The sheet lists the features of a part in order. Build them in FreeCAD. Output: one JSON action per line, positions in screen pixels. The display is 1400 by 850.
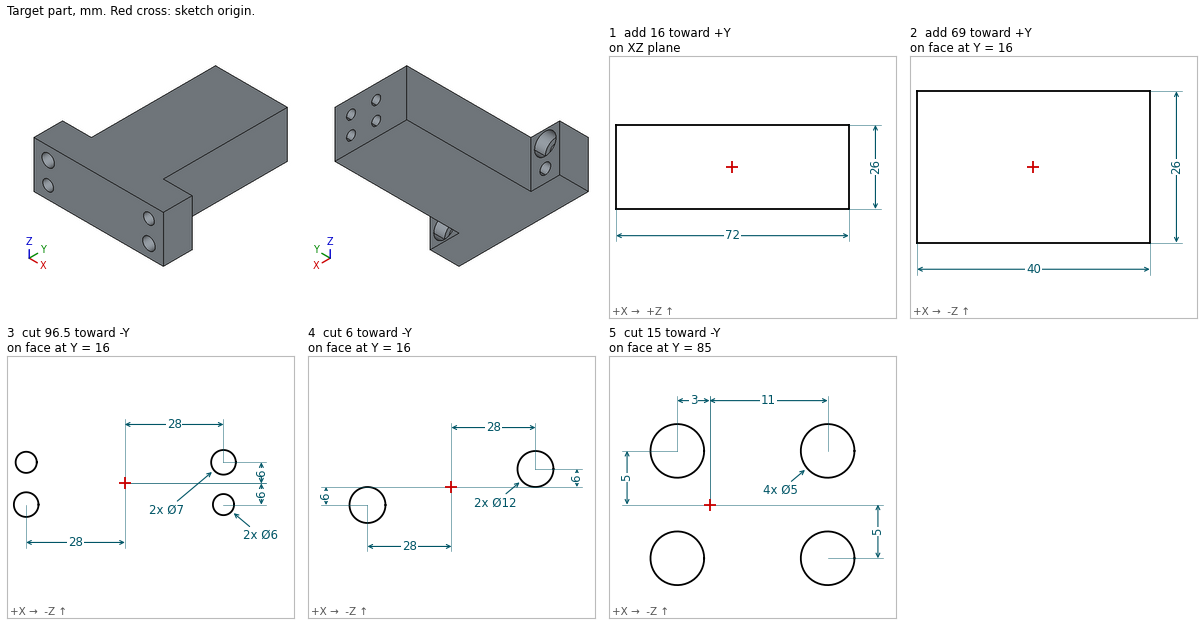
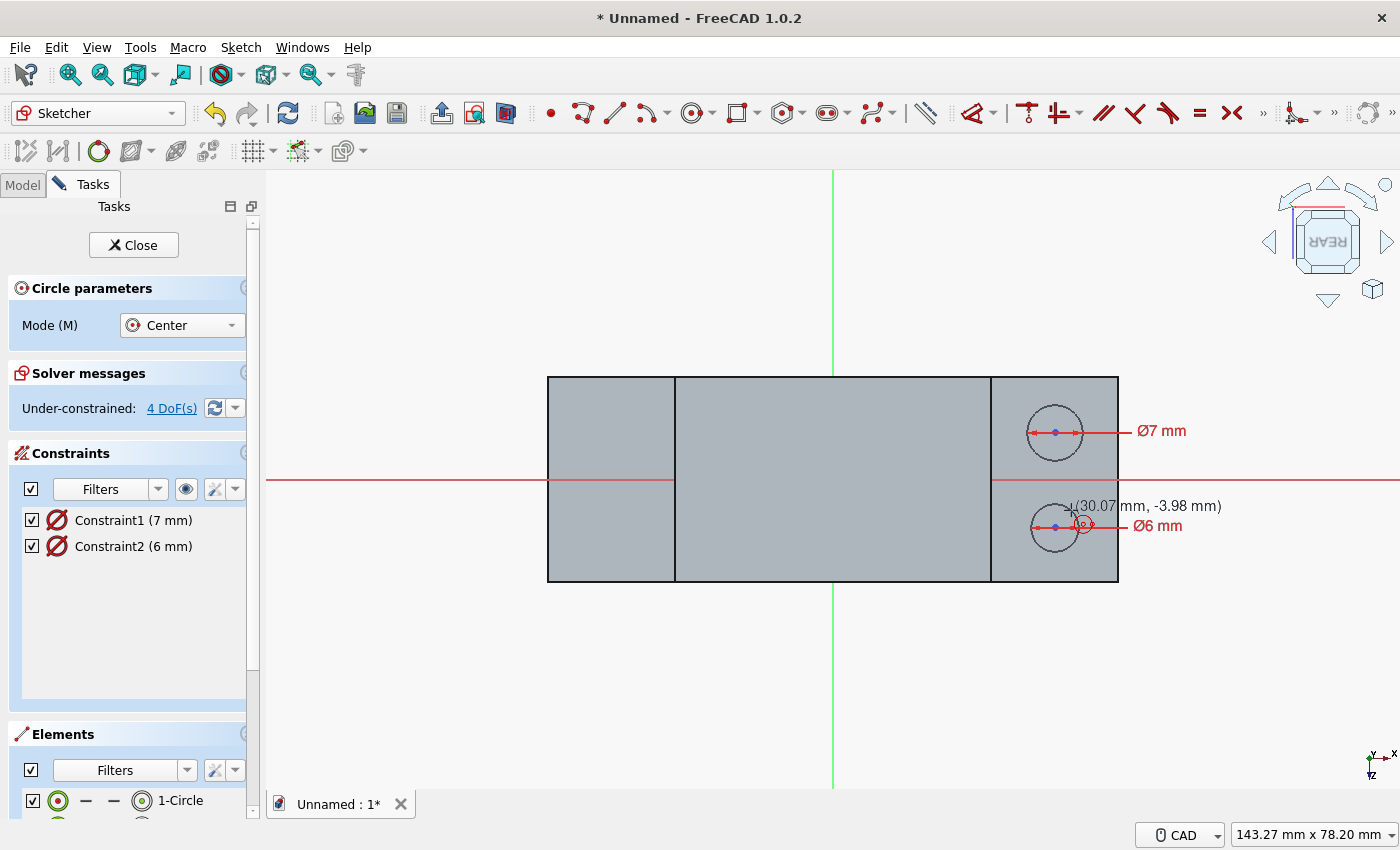
{"action": "left_click", "coordinate": [611, 527]}
{"action": "mouse_move", "coordinate": [631, 507]}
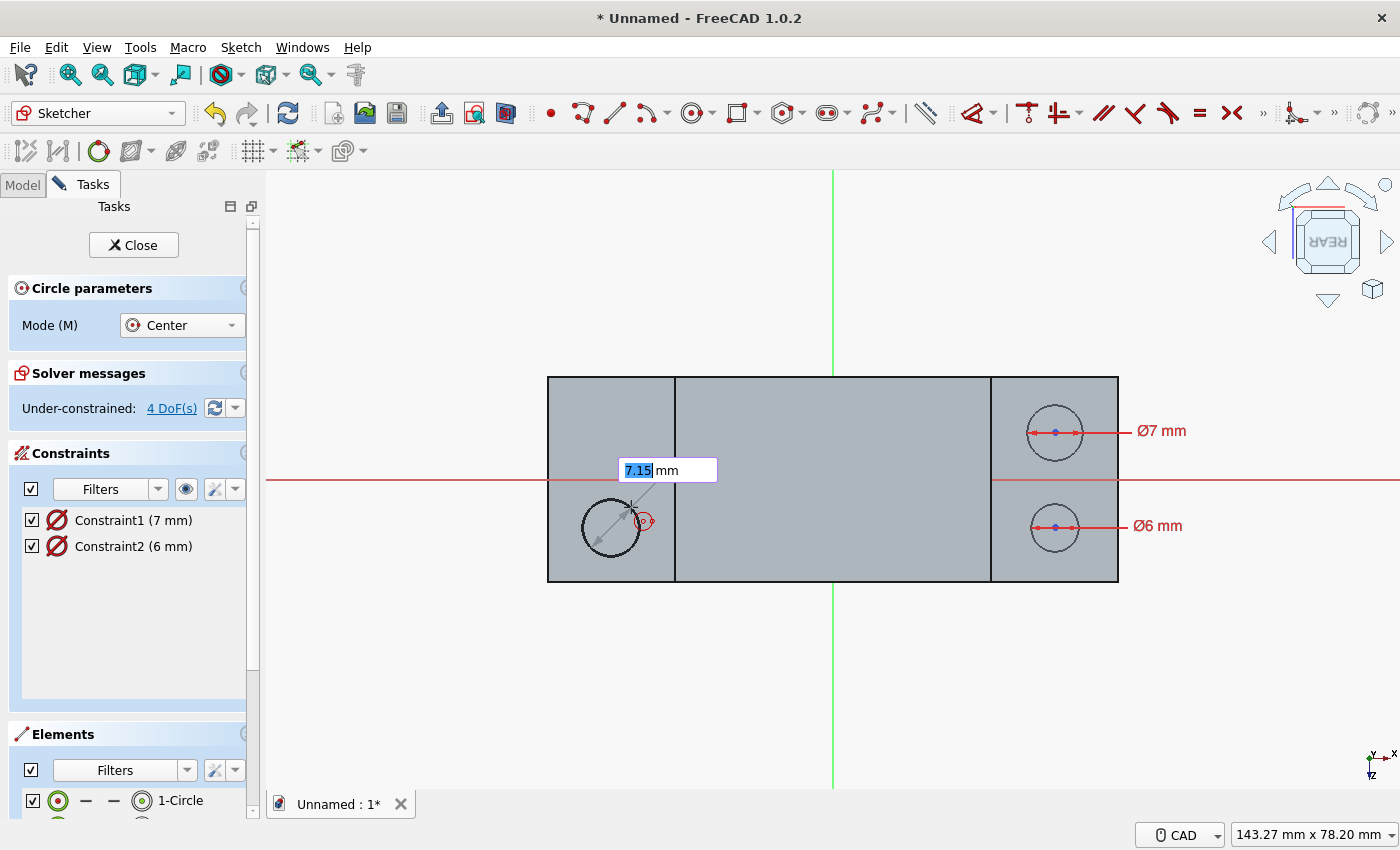
{"action": "type", "text": "7"}
{"action": "key", "text": "Return"}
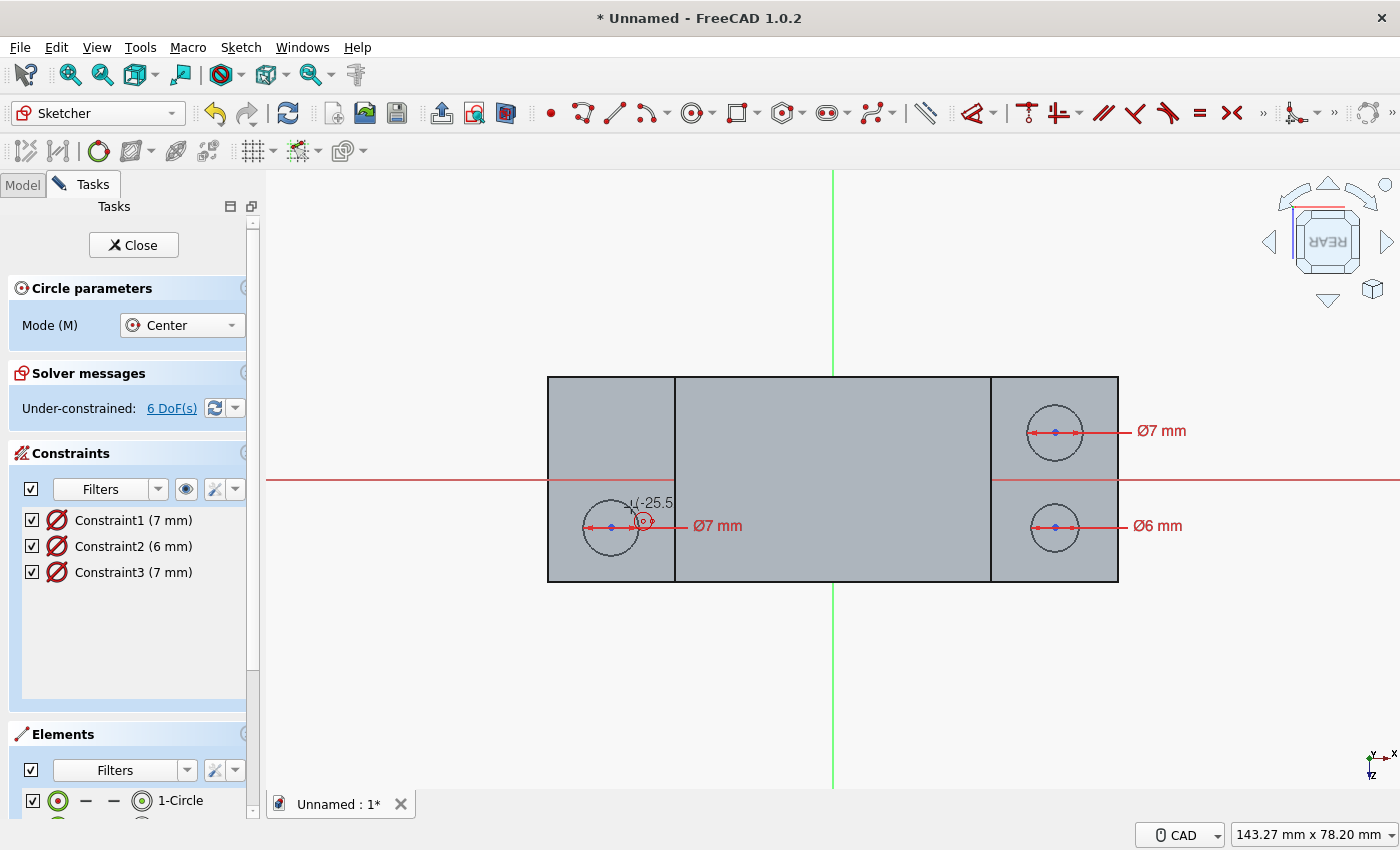
{"action": "left_click", "coordinate": [611, 432]}
{"action": "mouse_move", "coordinate": [628, 415]}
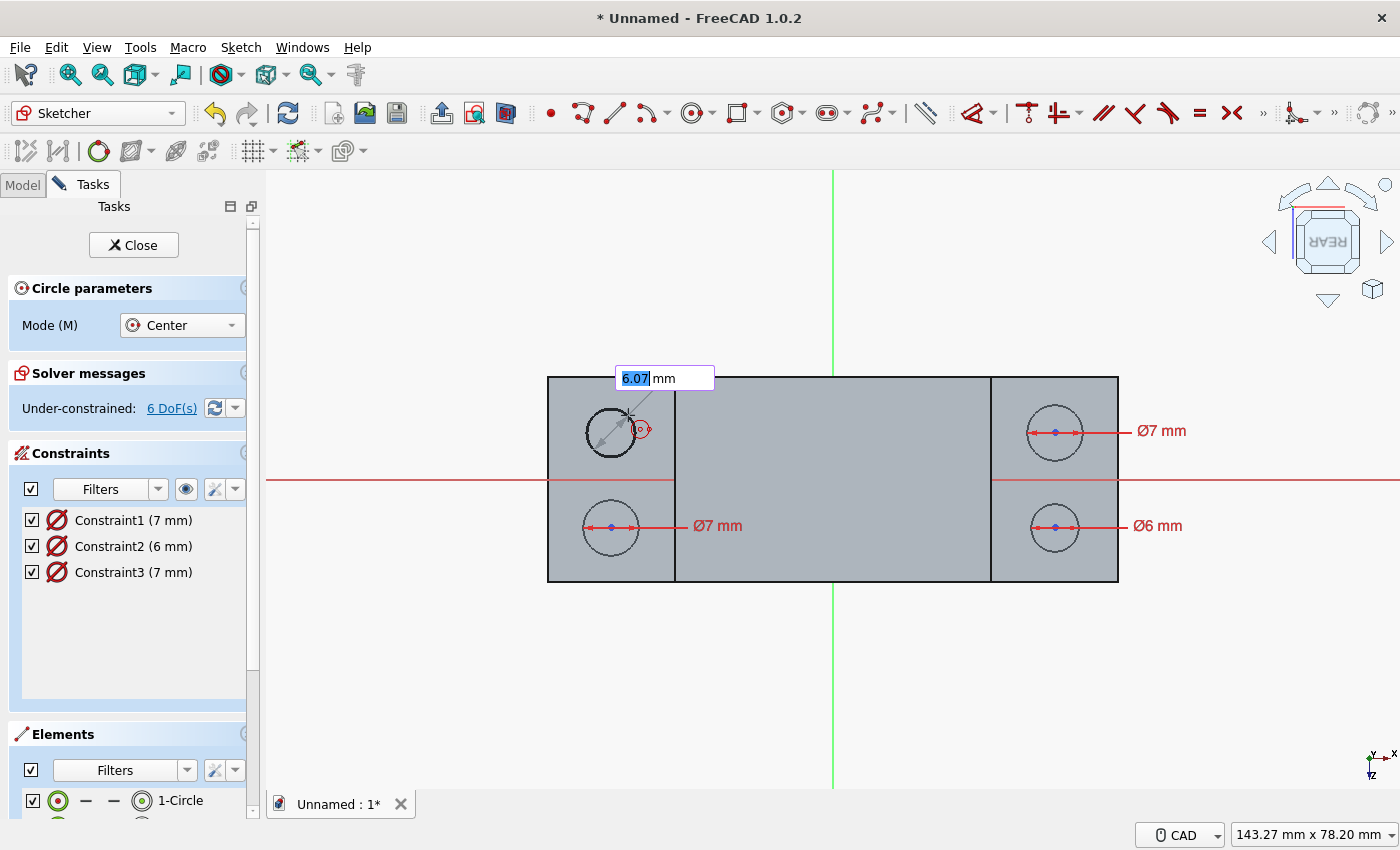
{"action": "type", "text": "6"}
{"action": "key", "text": "Return"}
{"action": "key", "text": "Escape"}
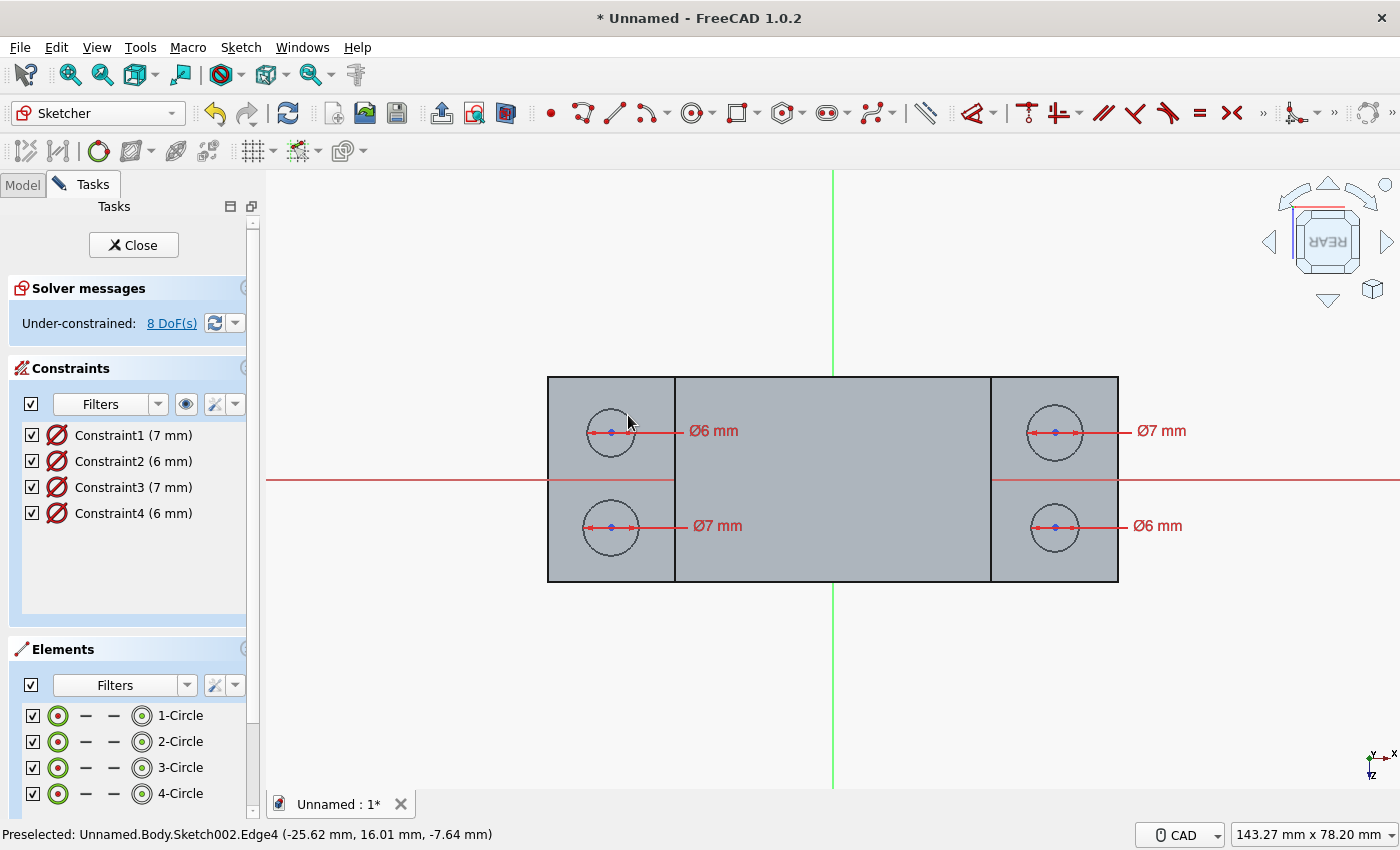
{"action": "left_click", "coordinate": [1055, 433]}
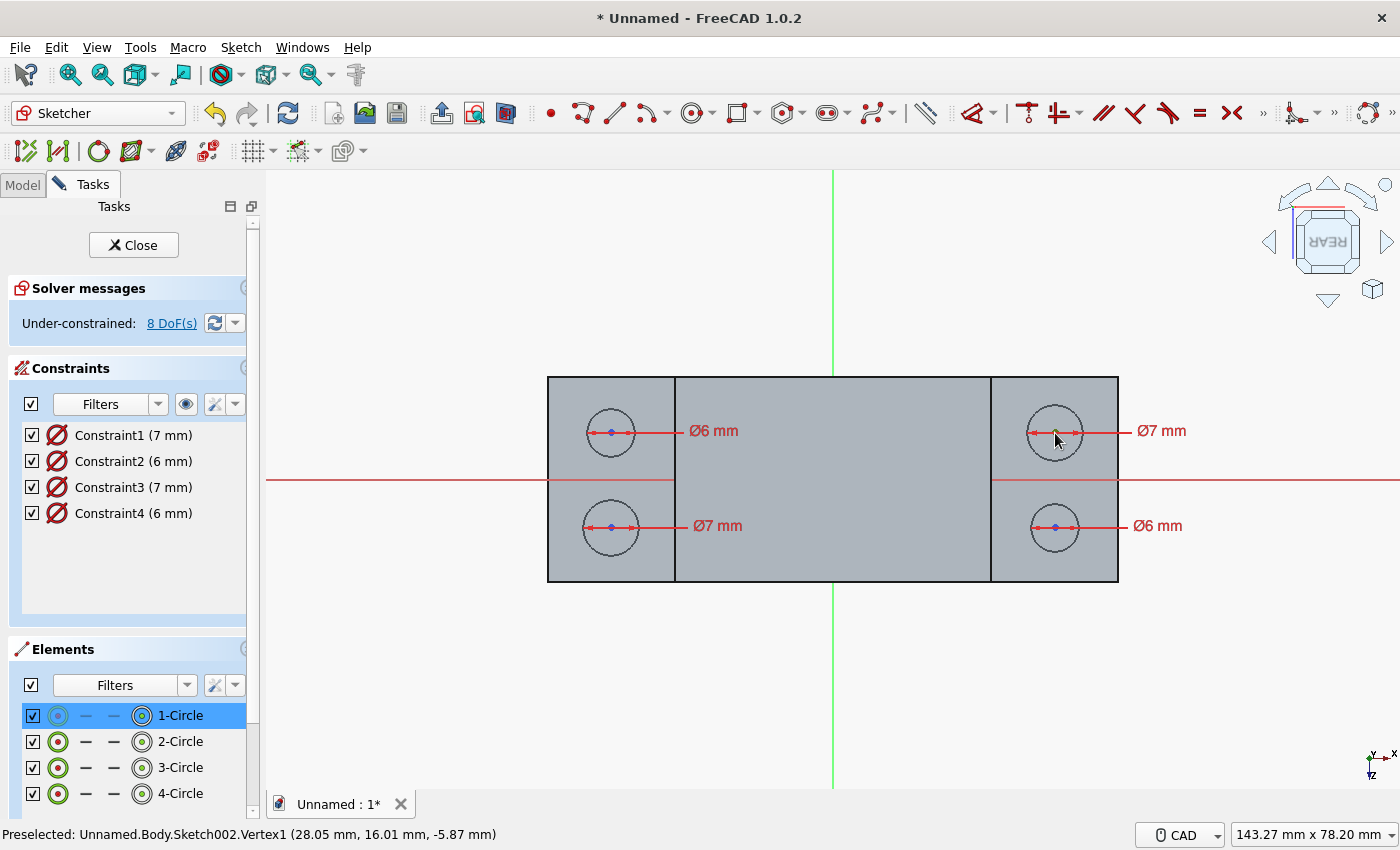
{"action": "left_click", "coordinate": [1055, 528]}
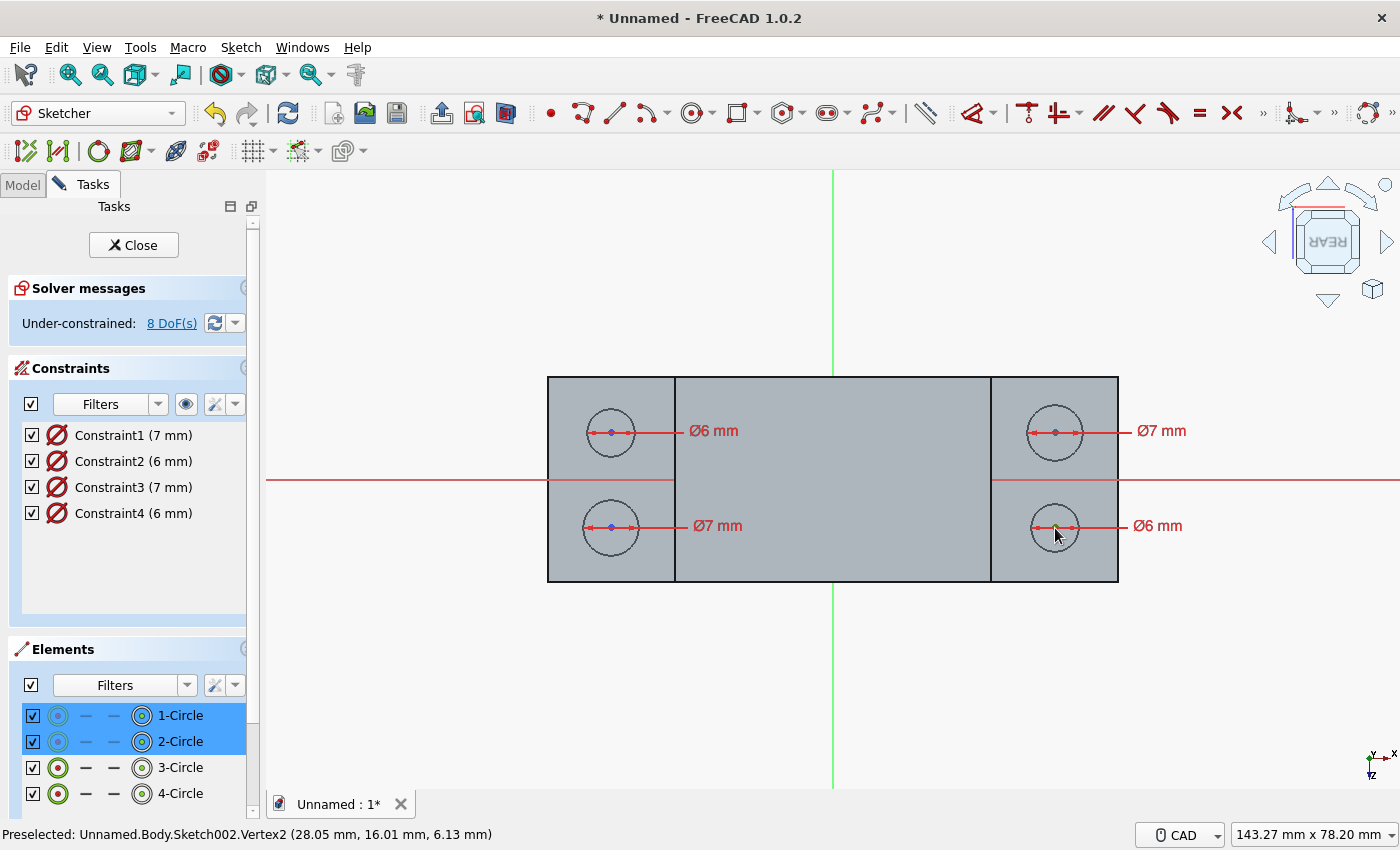
{"action": "key", "text": "v"}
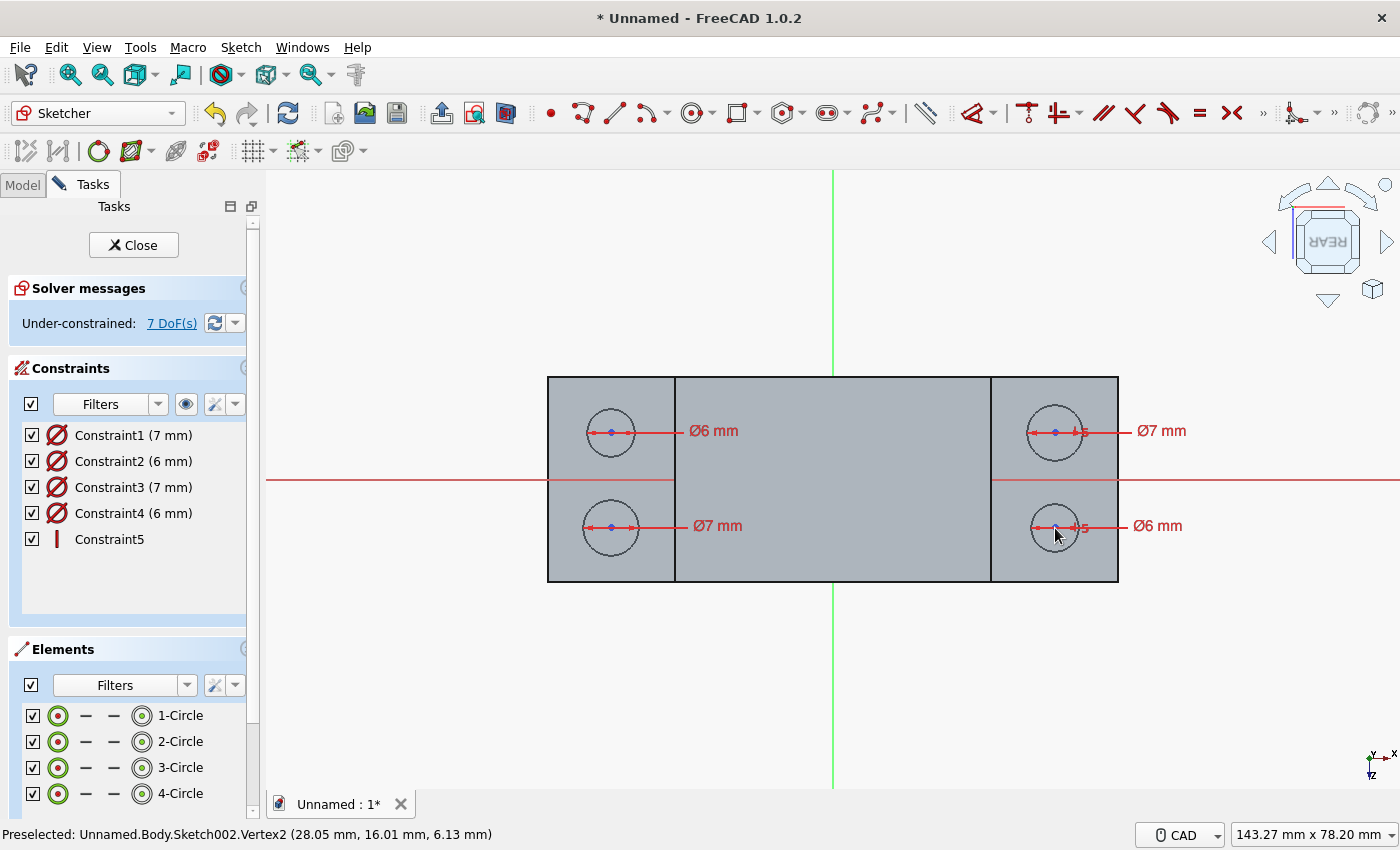
{"action": "left_click", "coordinate": [1055, 528]}